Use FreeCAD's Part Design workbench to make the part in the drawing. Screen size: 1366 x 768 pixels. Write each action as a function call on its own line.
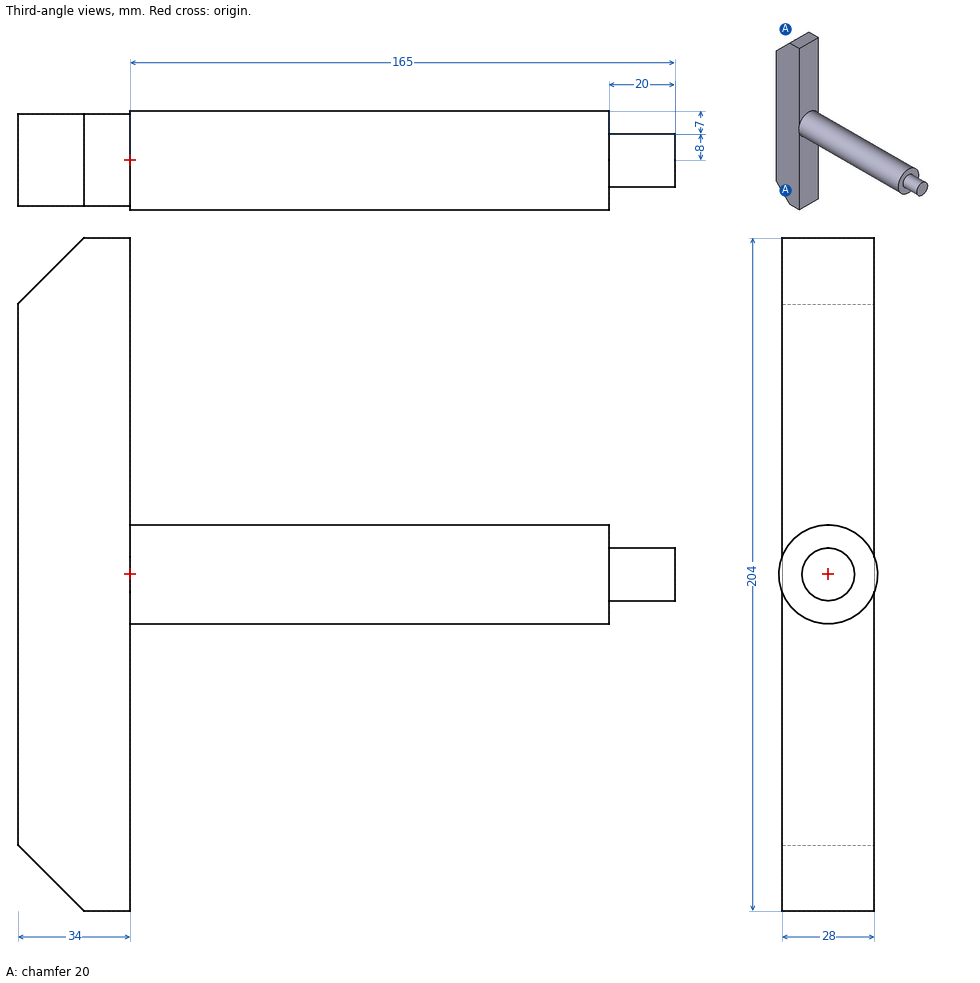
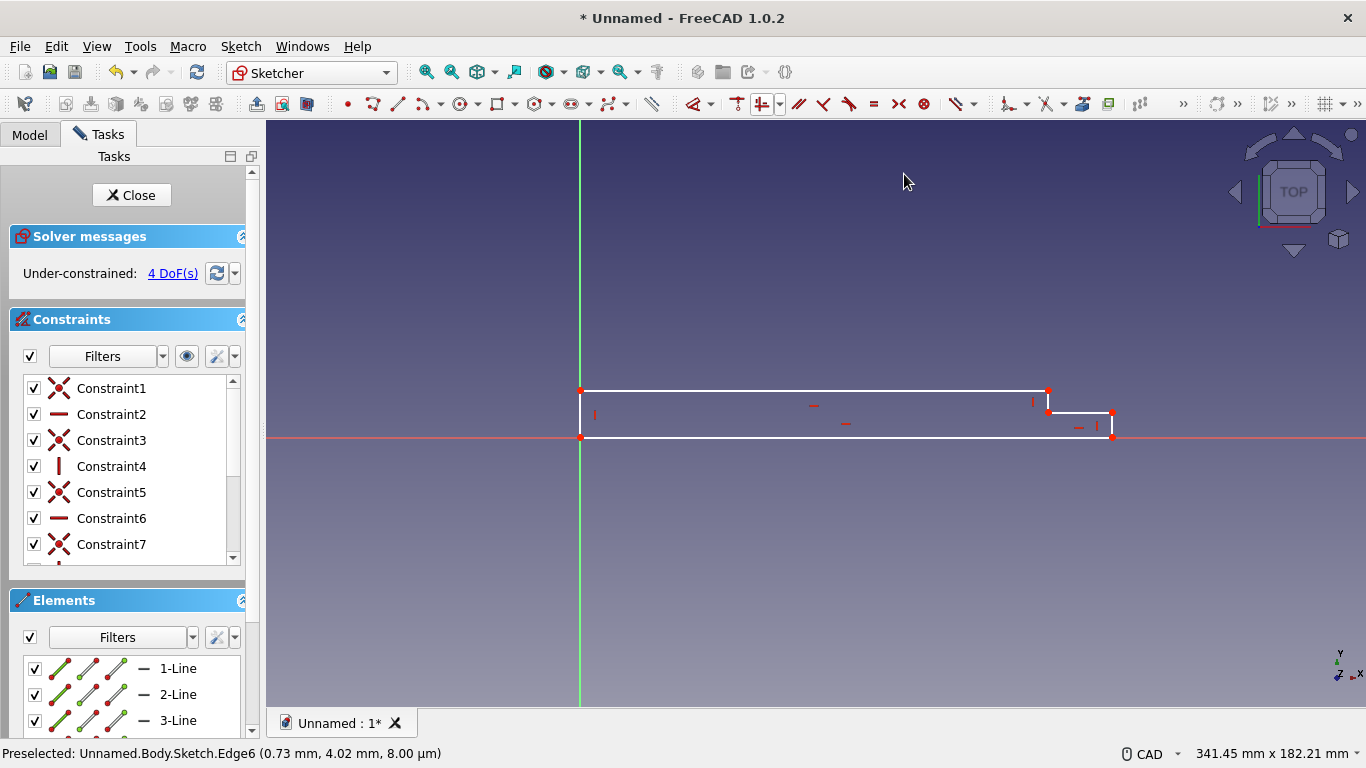
click(692, 104)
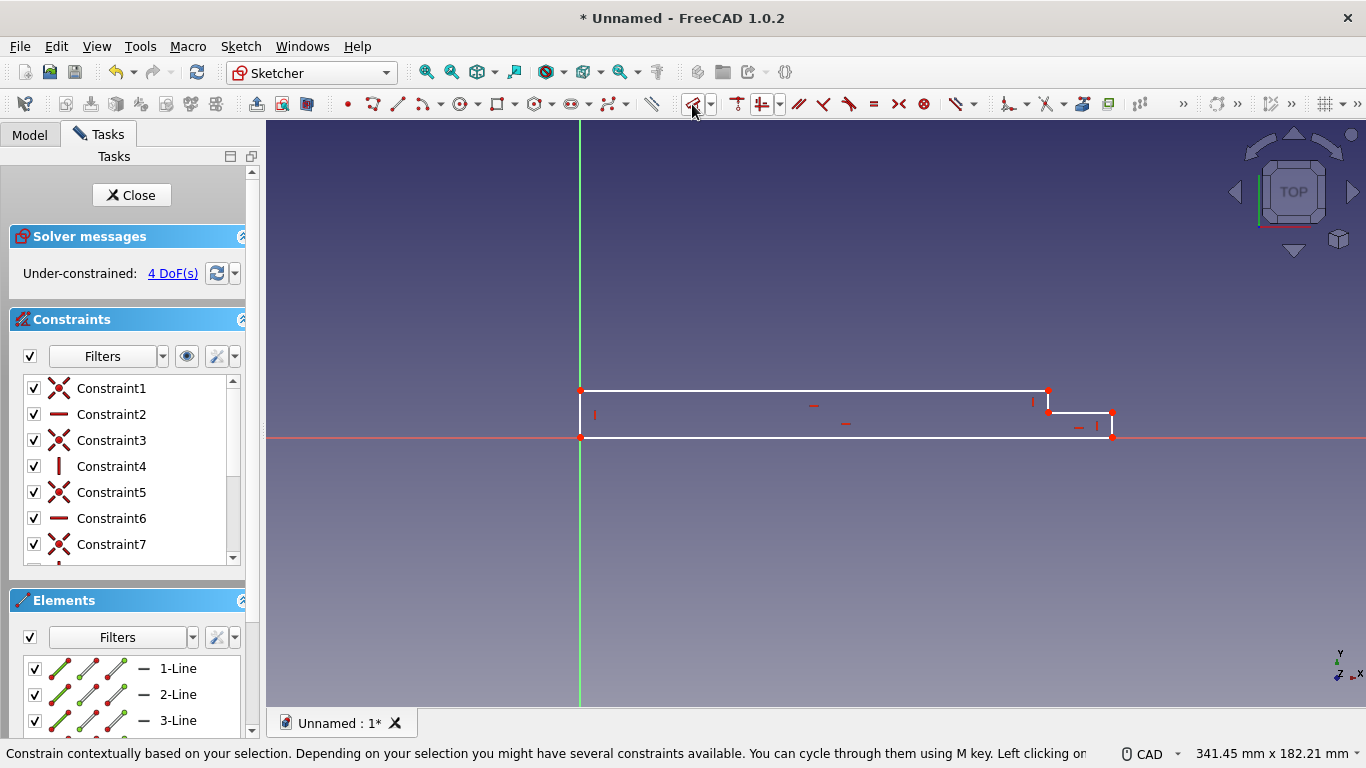
scroll(1112, 428, up, 3)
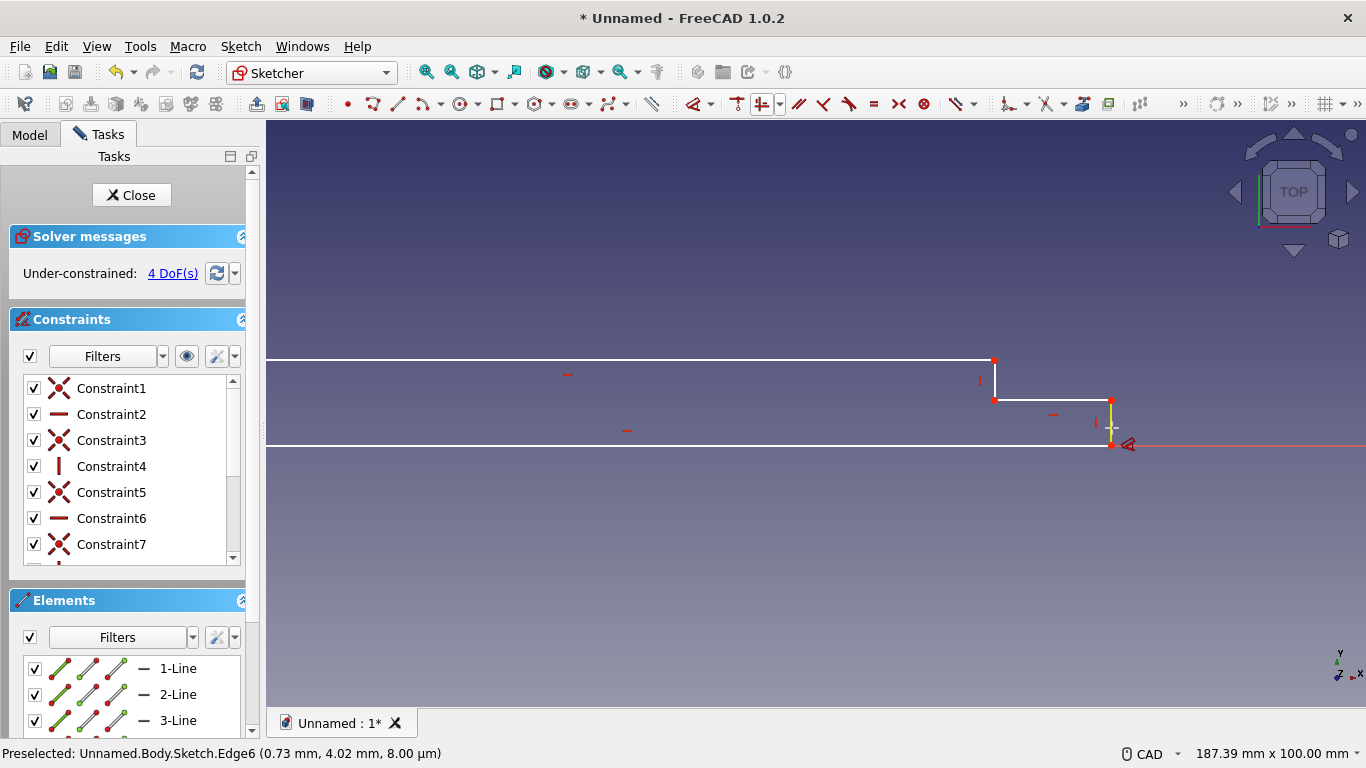
click(1111, 427)
click(1145, 423)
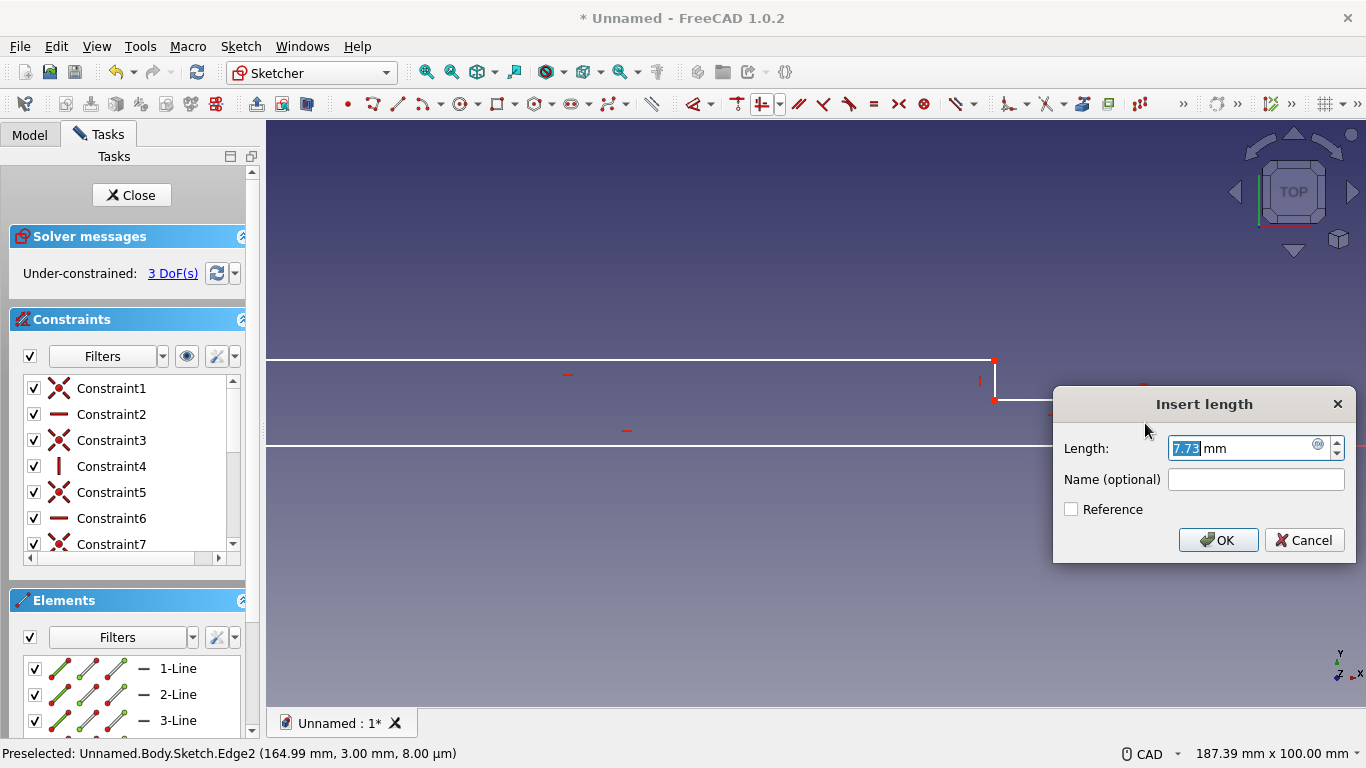
text(8)
key(Return)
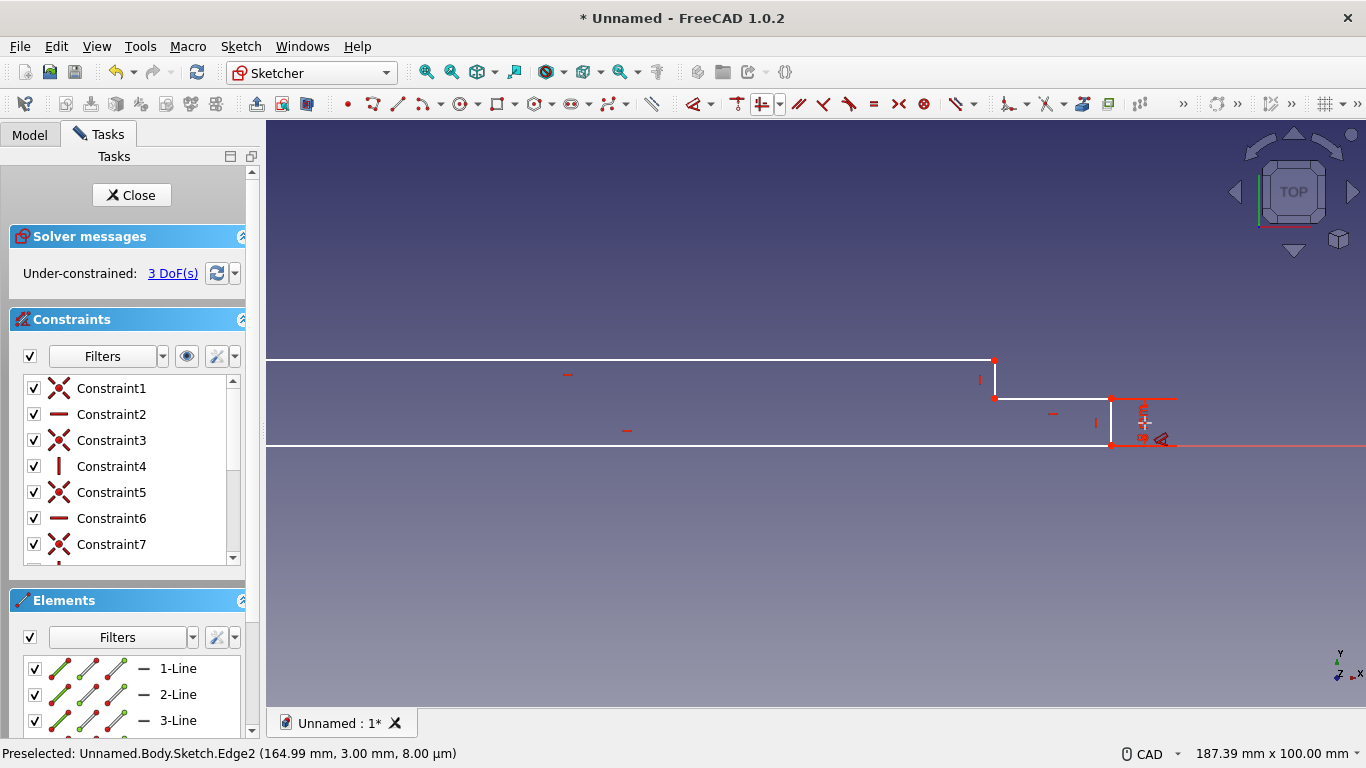
click(995, 387)
click(1029, 379)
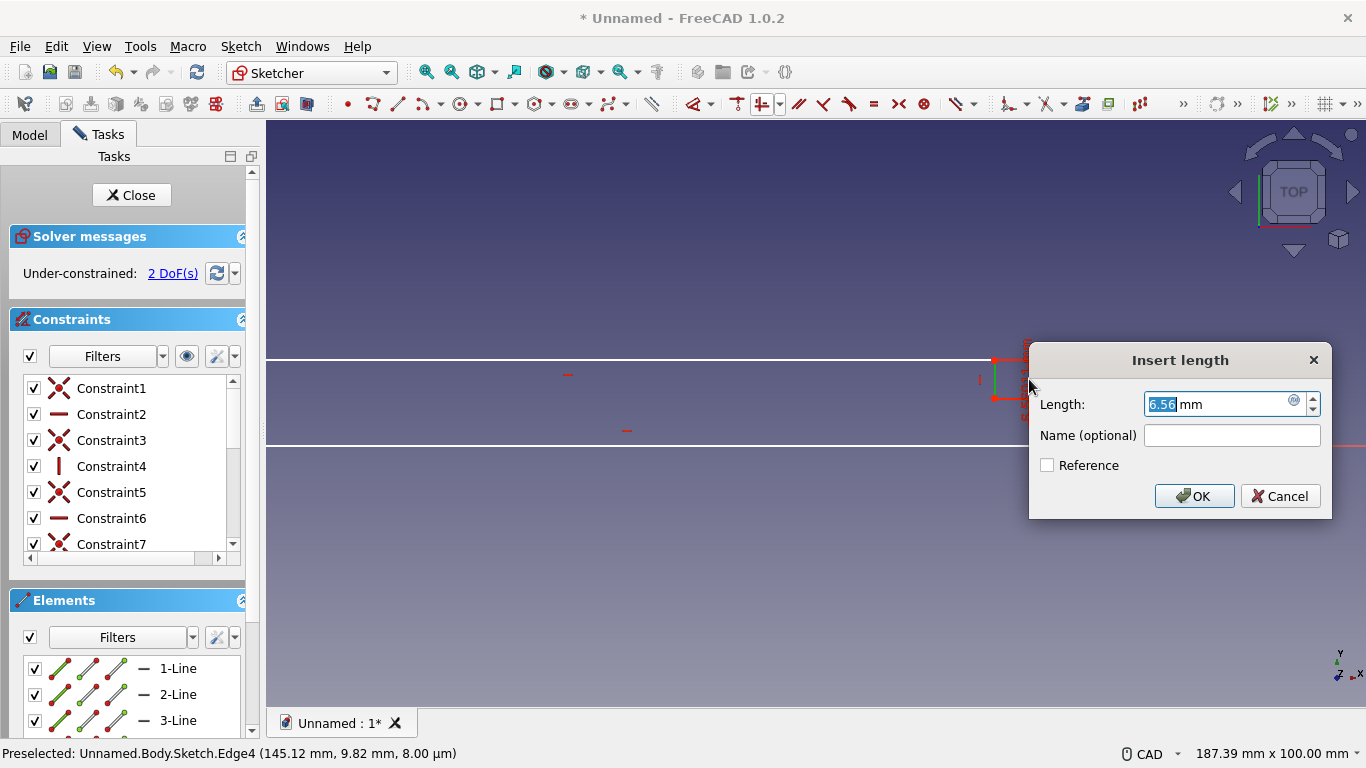
text(7)
key(Return)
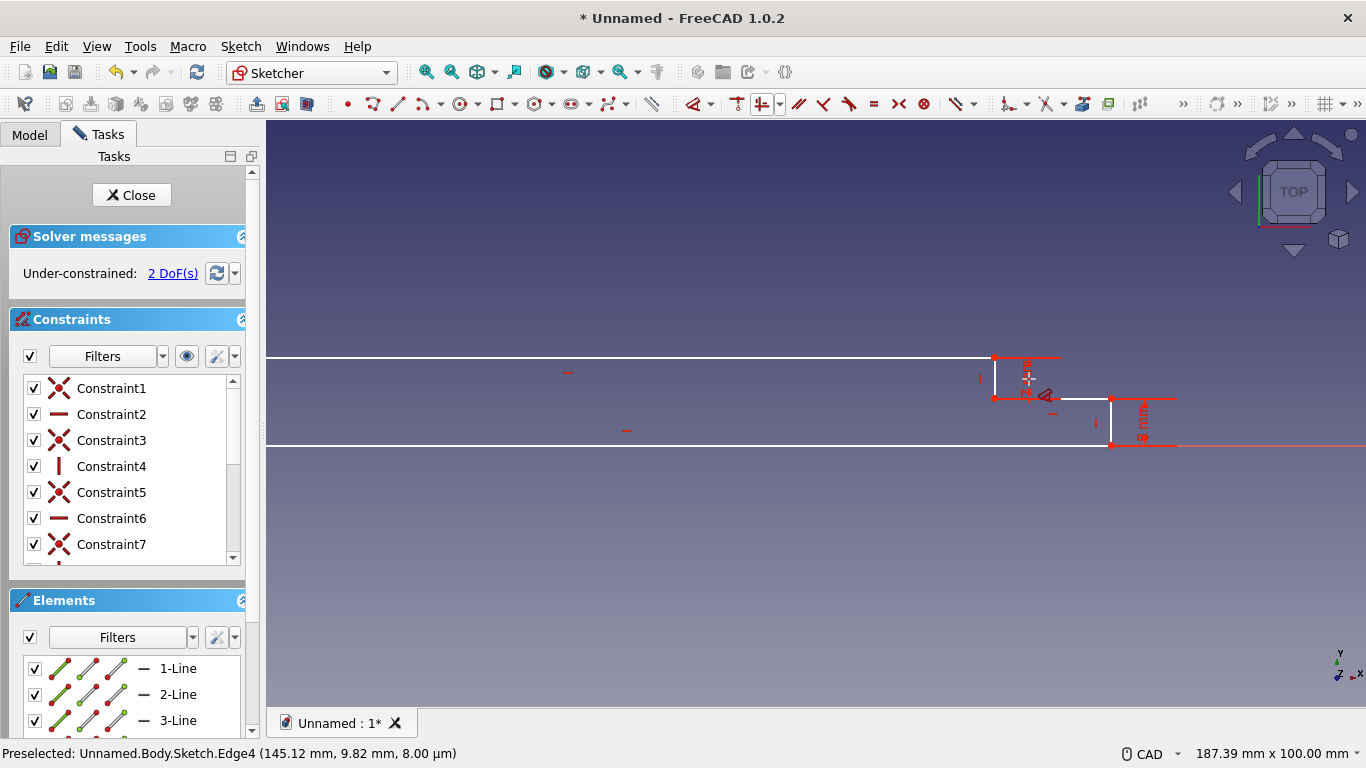
click(1076, 399)
click(1053, 341)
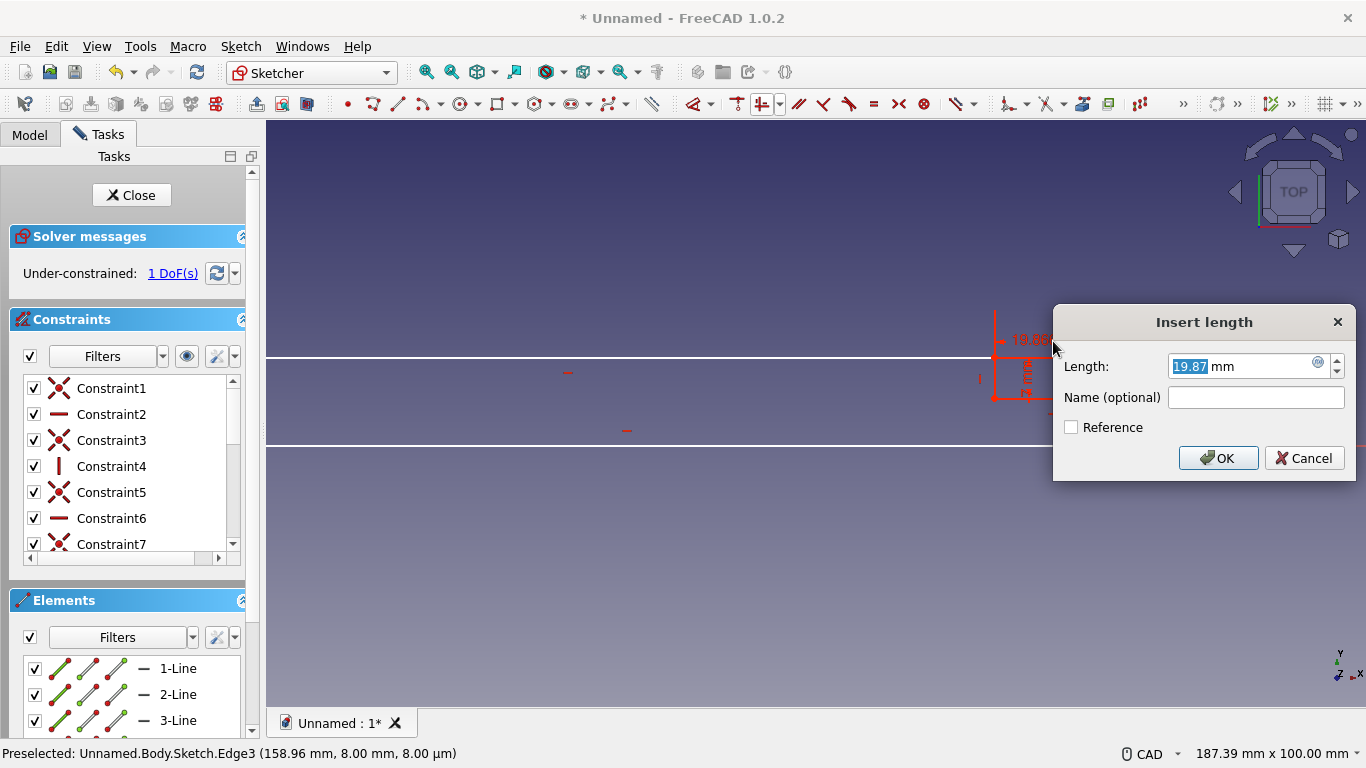
text(20)
key(Return)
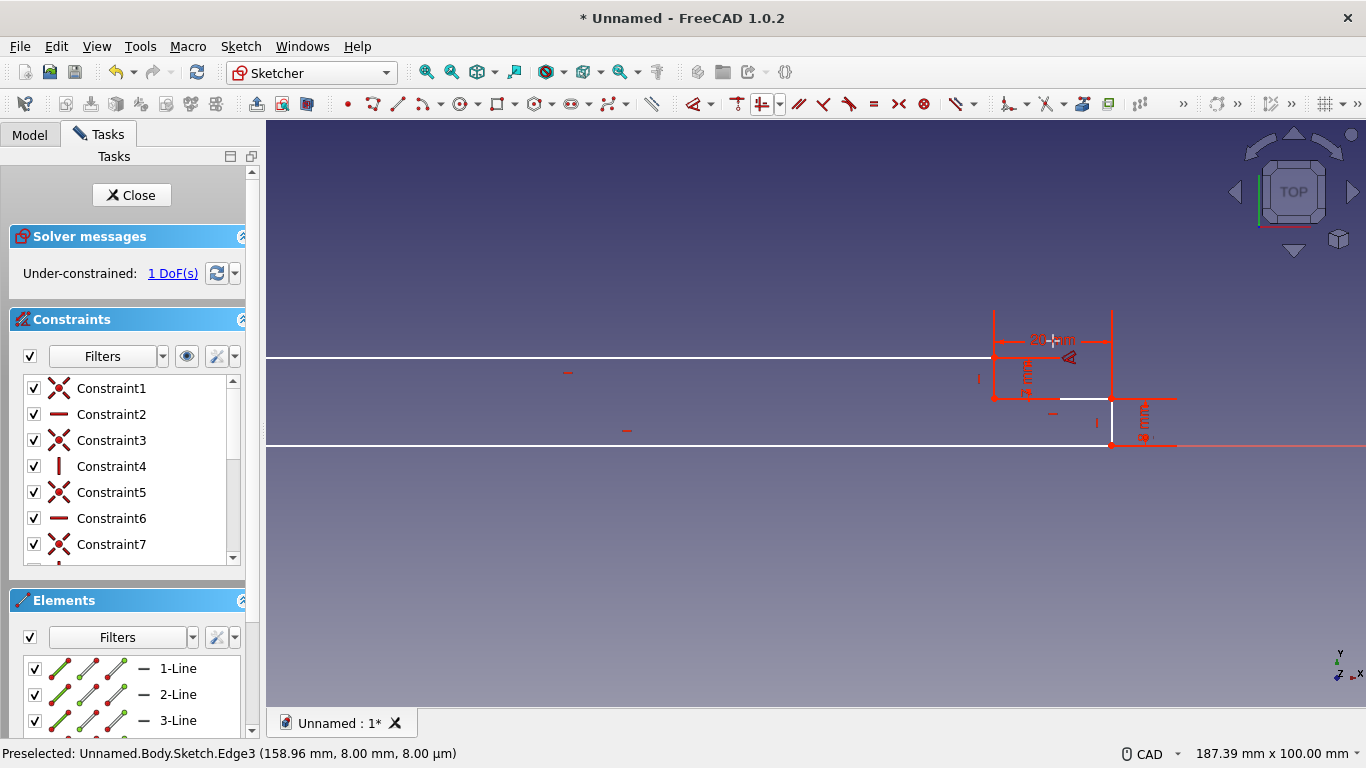
click(434, 446)
click(703, 480)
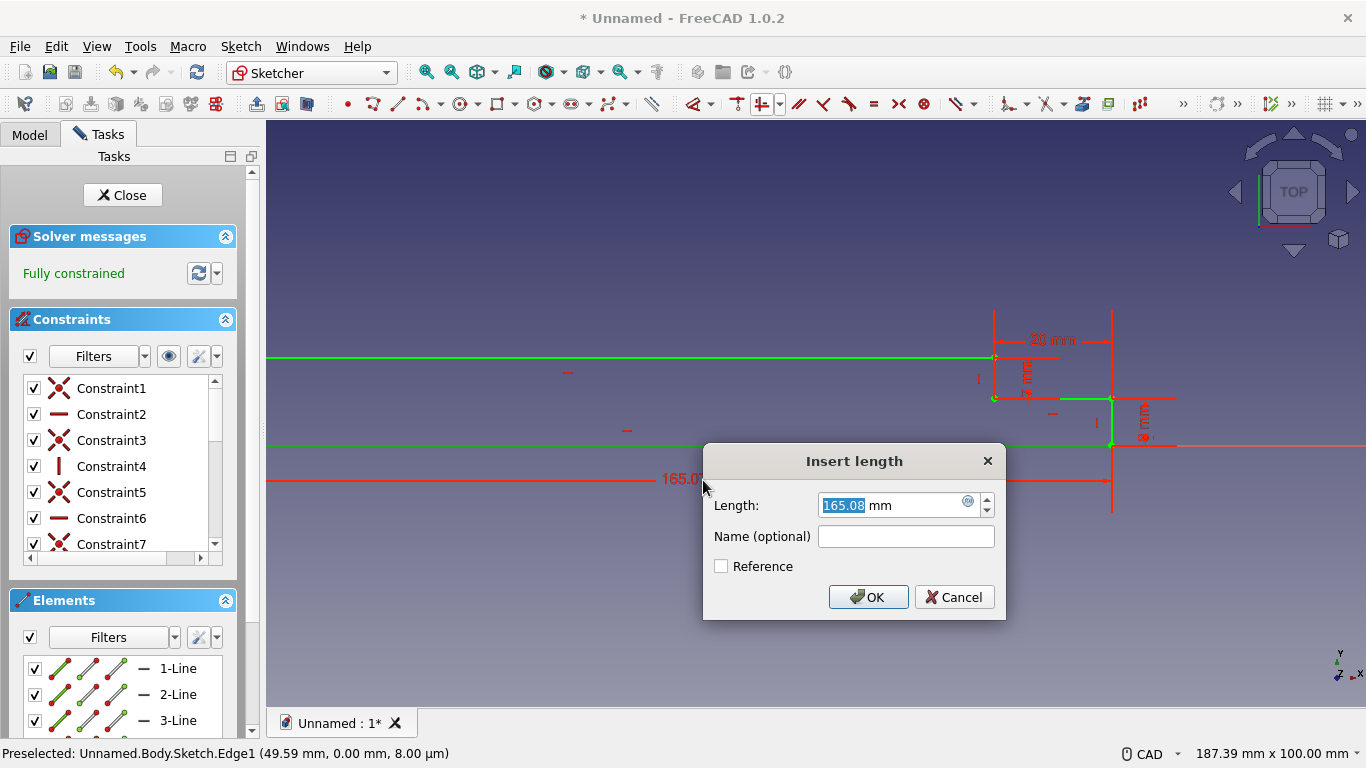
text(165)
key(Return)
key(Escape)